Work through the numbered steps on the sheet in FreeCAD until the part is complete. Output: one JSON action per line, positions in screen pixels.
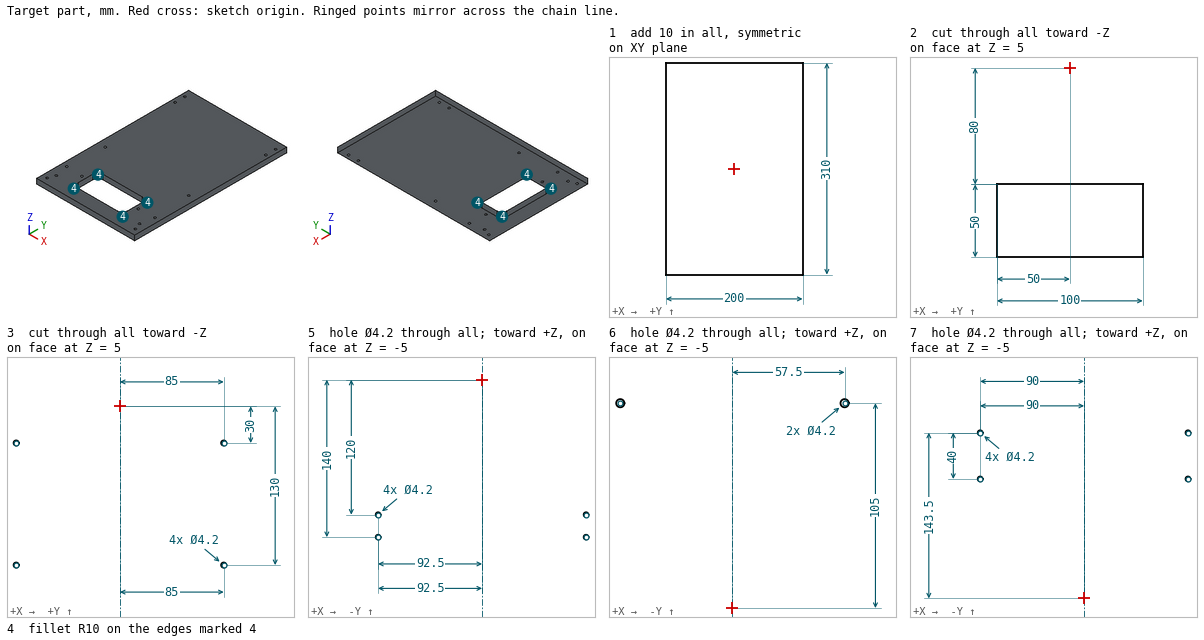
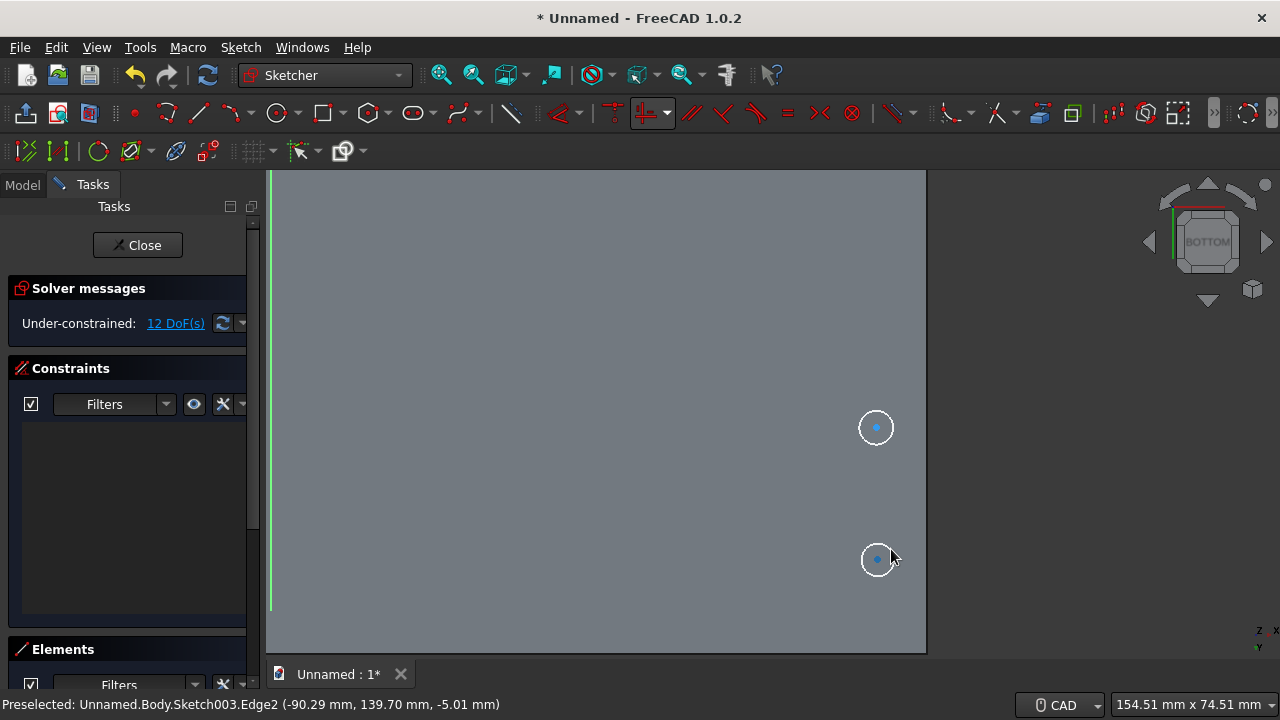
{"action": "left_click", "coordinate": [889, 548]}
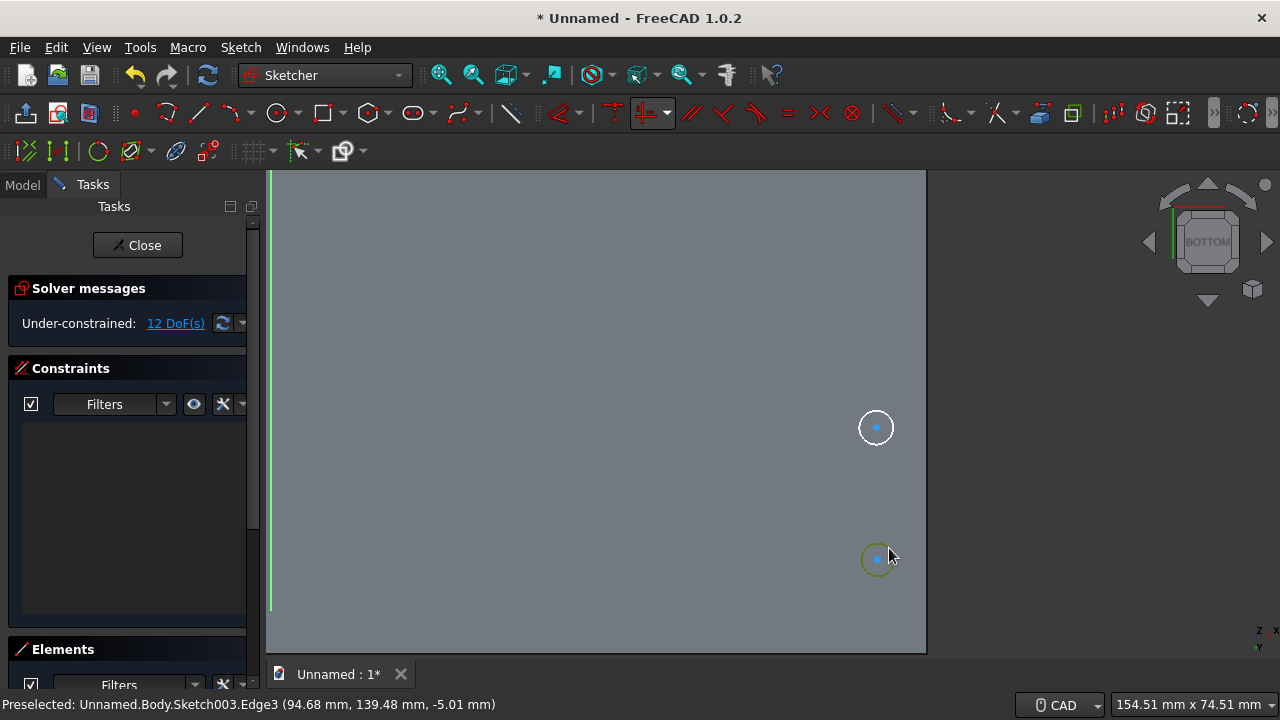
{"action": "left_click", "coordinate": [888, 416]}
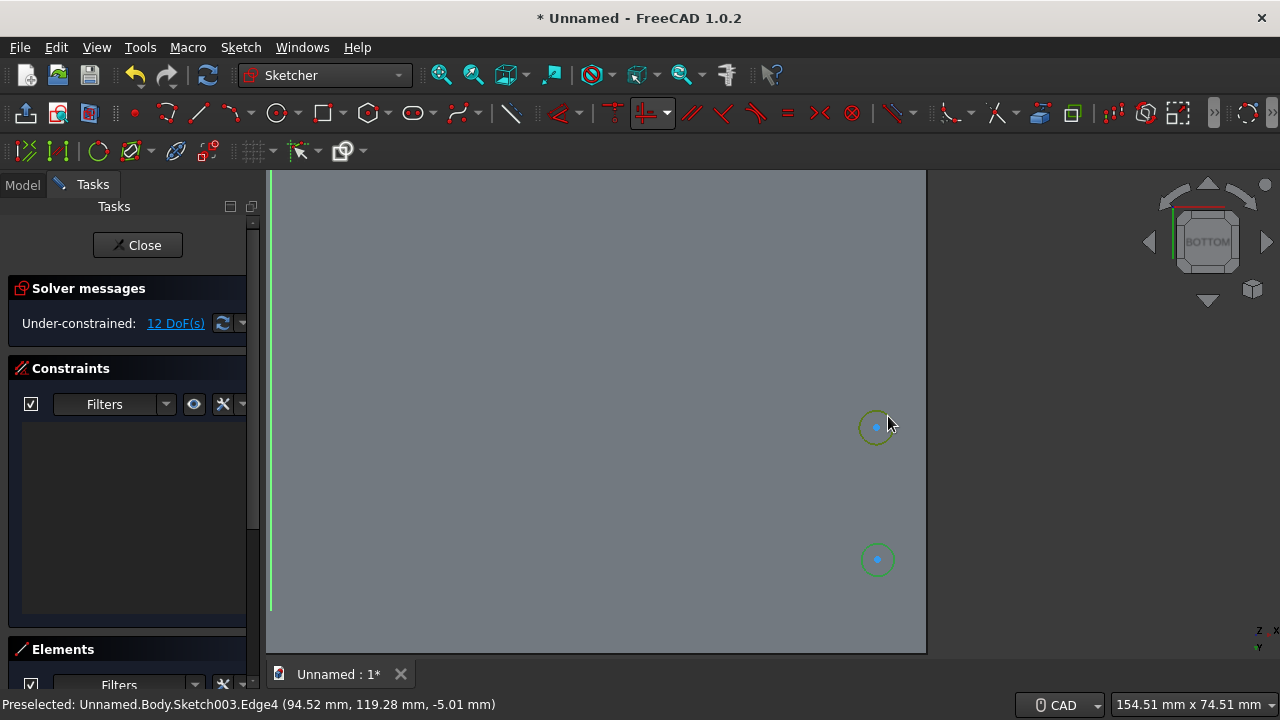
{"action": "left_click", "coordinate": [788, 114]}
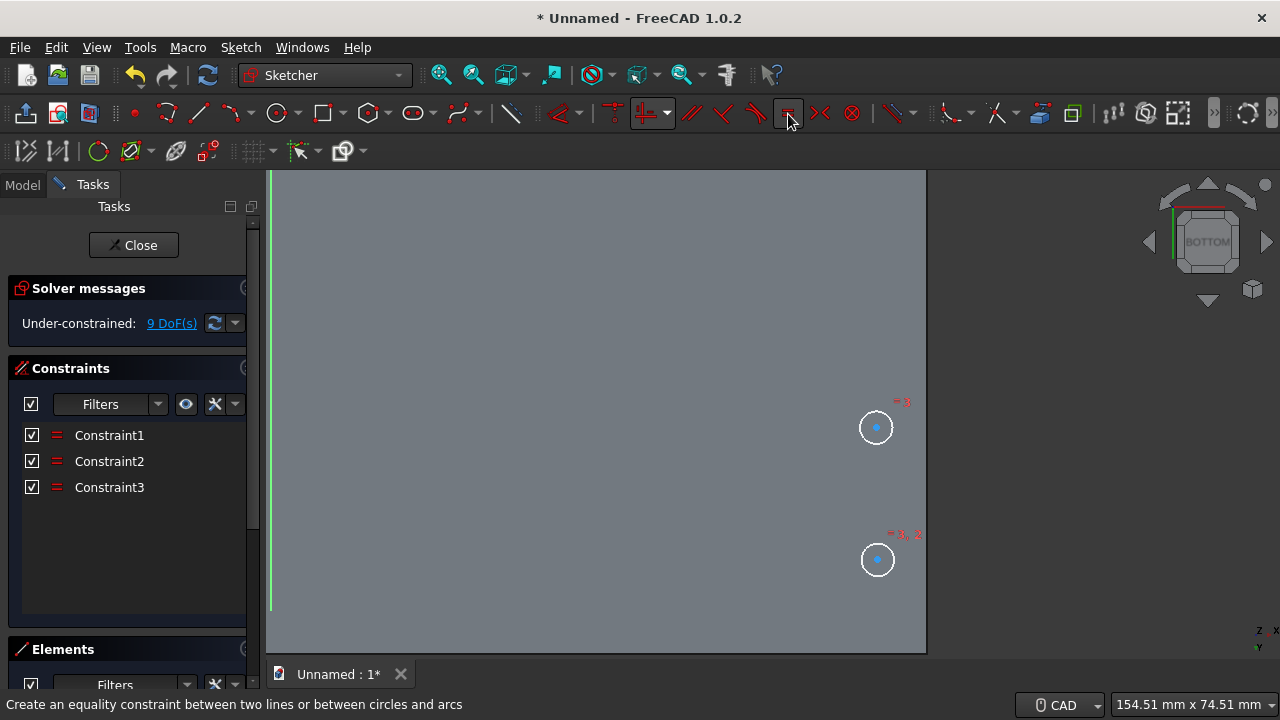
{"action": "scroll", "coordinate": [891, 549], "scroll_direction": "down", "scroll_amount": 6}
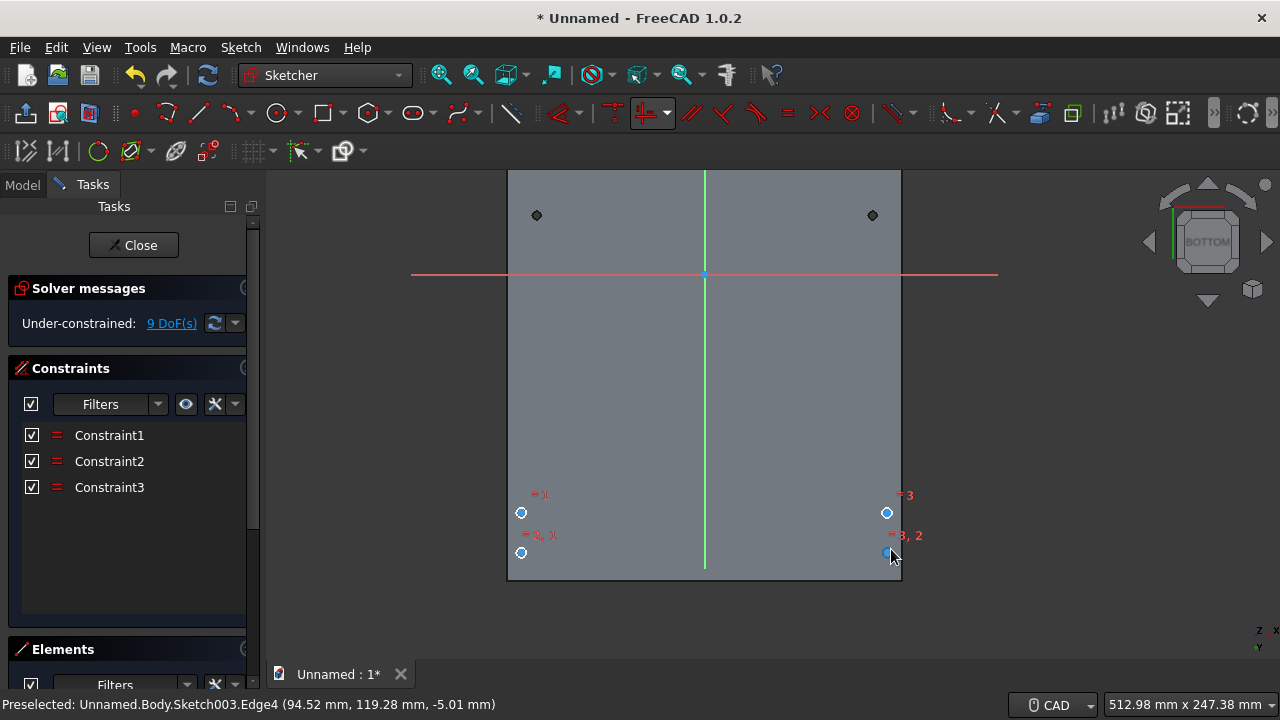
{"action": "left_click", "coordinate": [521, 553]}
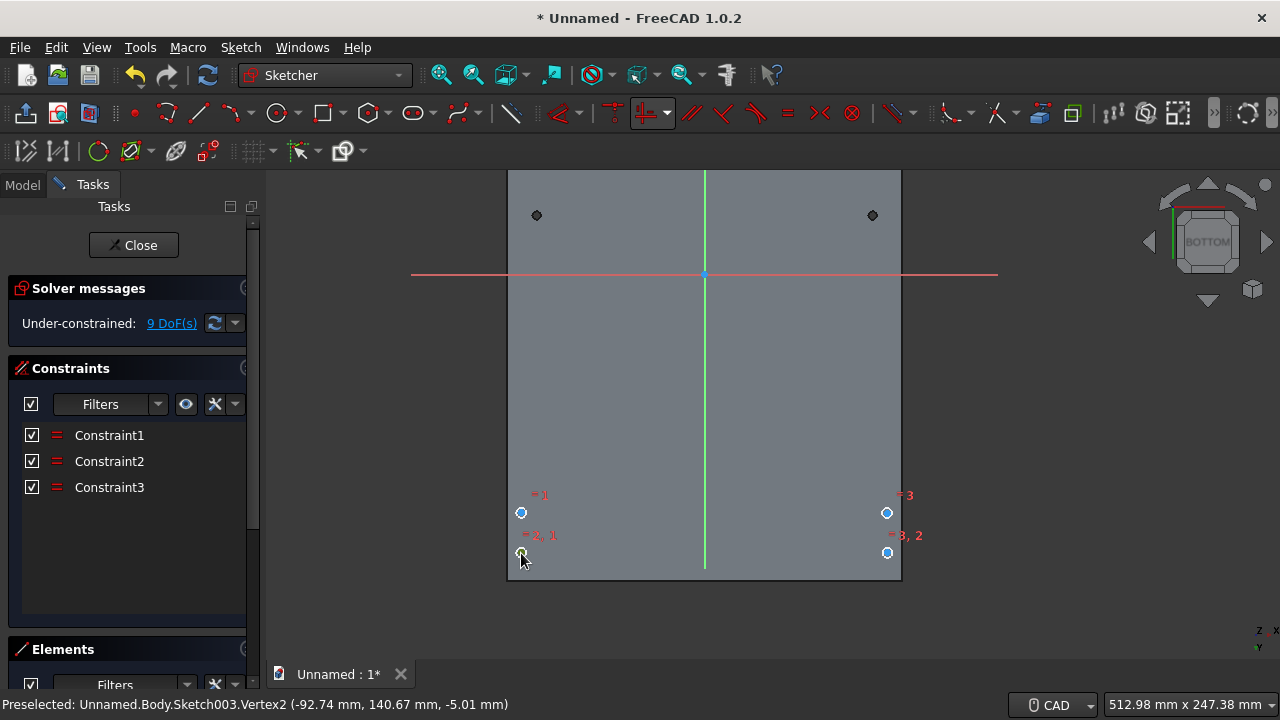
{"action": "left_click", "coordinate": [887, 553]}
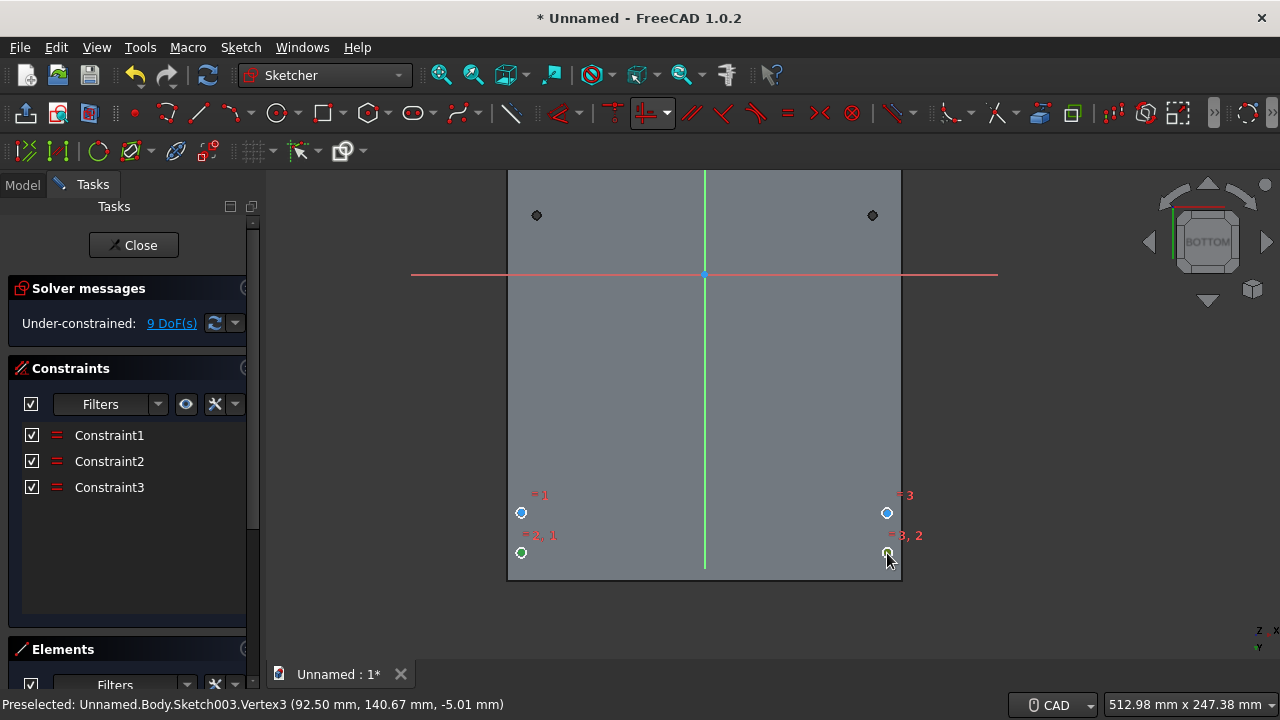
{"action": "left_click", "coordinate": [705, 569]}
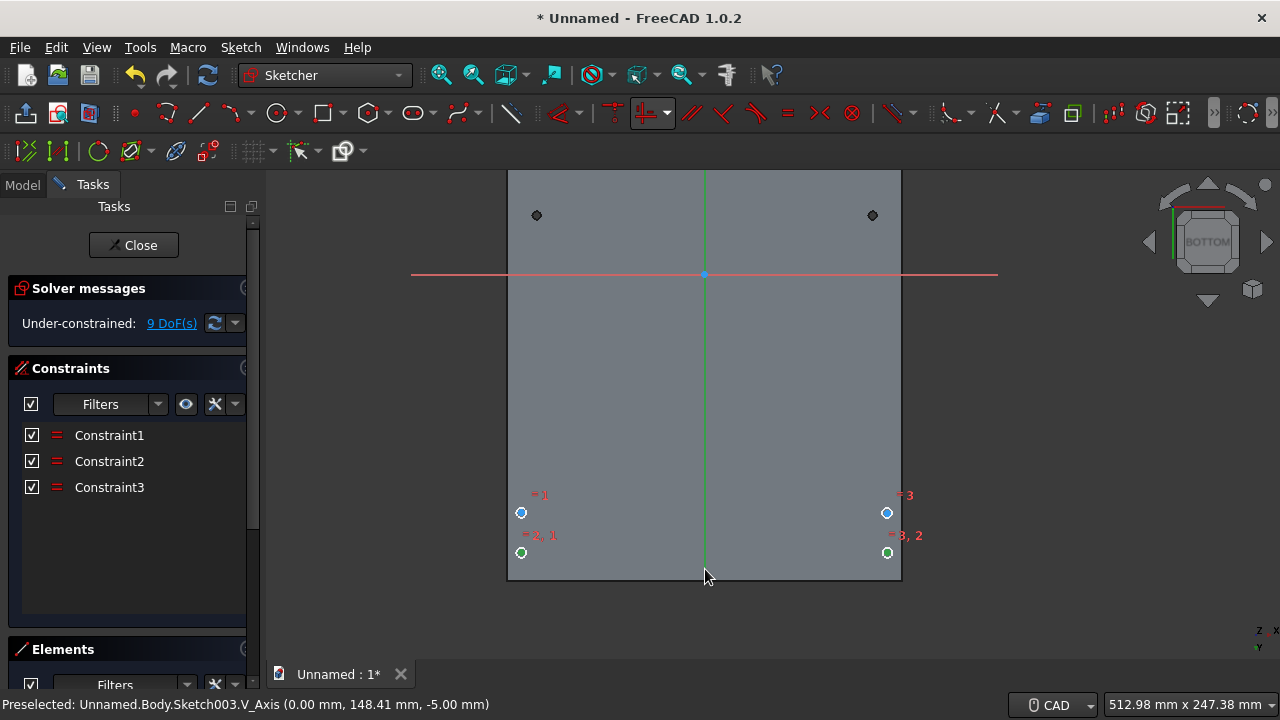
{"action": "left_click", "coordinate": [820, 114]}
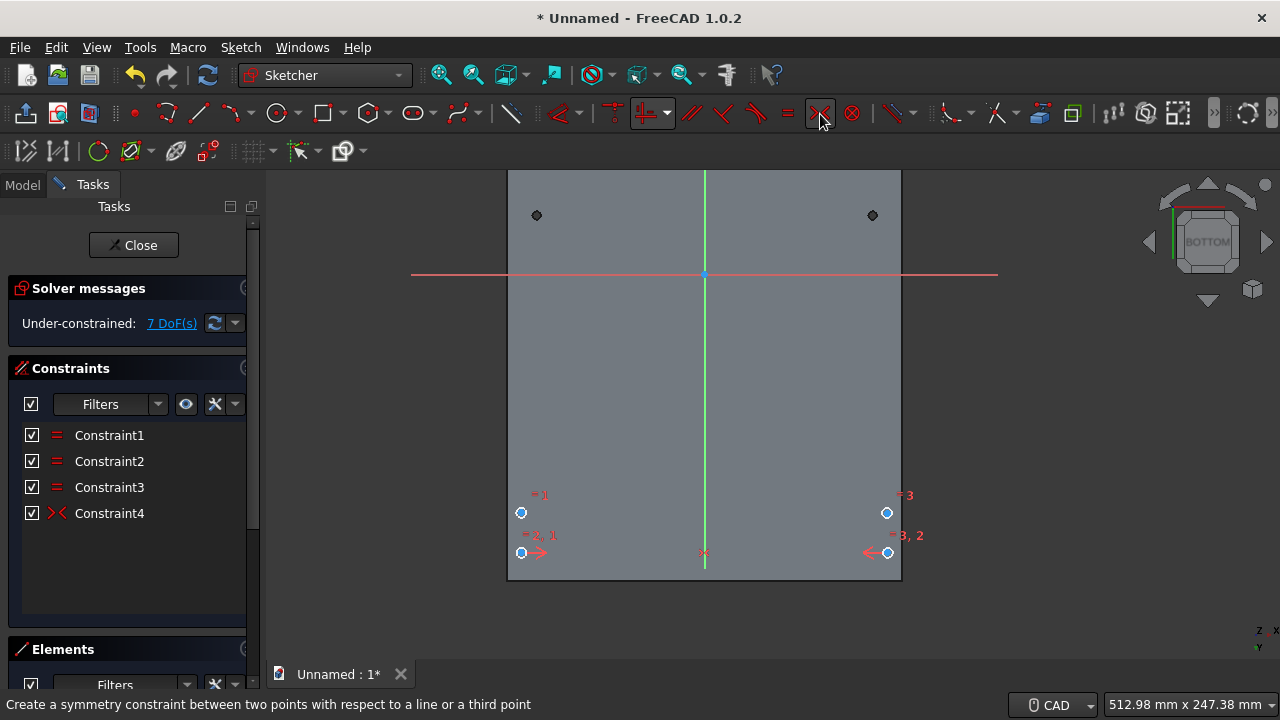
{"action": "left_click", "coordinate": [521, 513]}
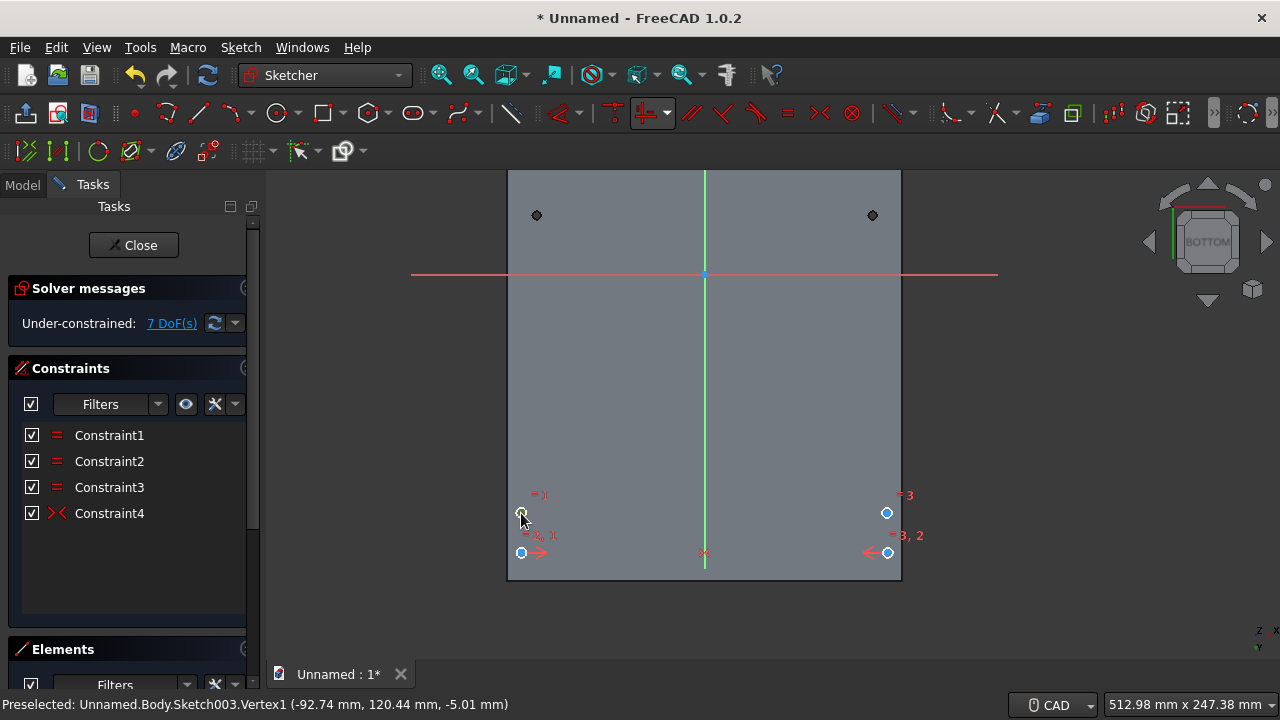
{"action": "left_click", "coordinate": [887, 513]}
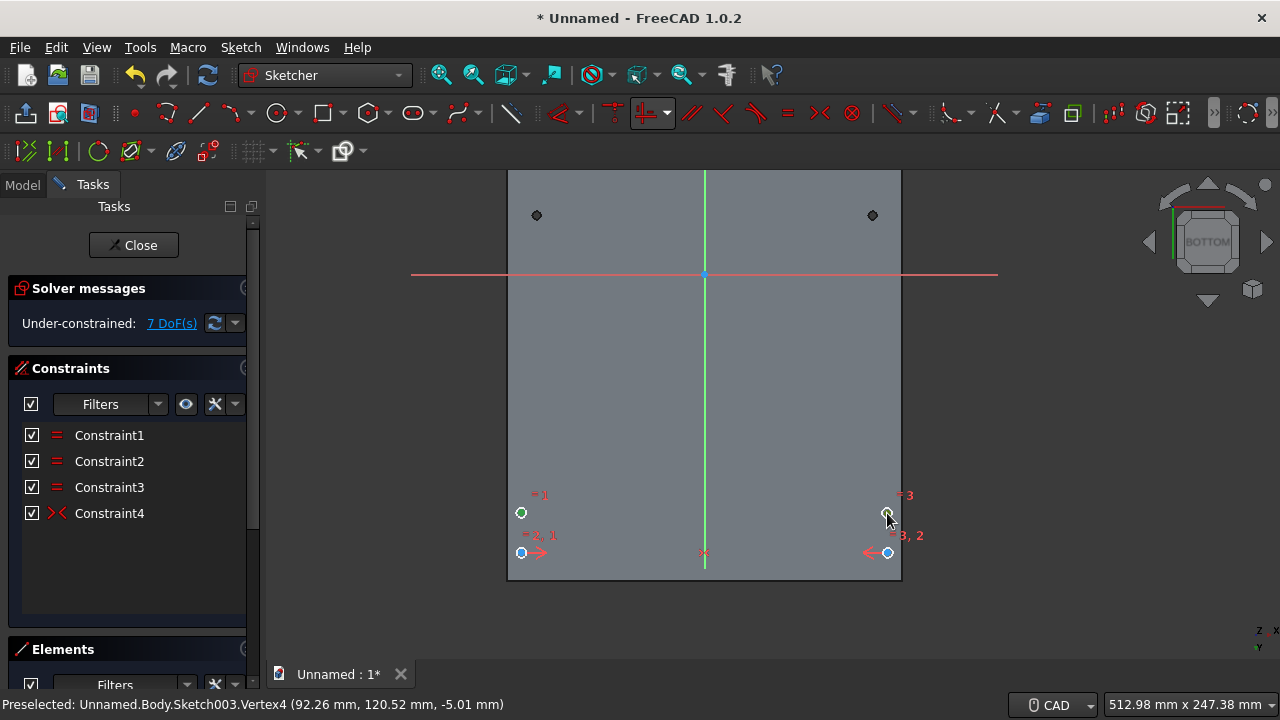
{"action": "left_click", "coordinate": [705, 569]}